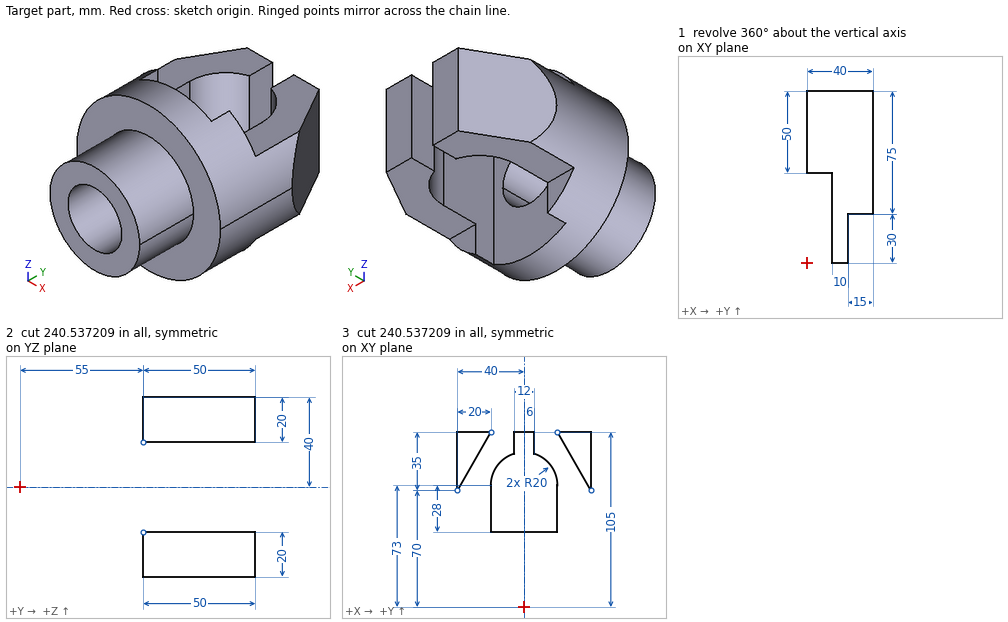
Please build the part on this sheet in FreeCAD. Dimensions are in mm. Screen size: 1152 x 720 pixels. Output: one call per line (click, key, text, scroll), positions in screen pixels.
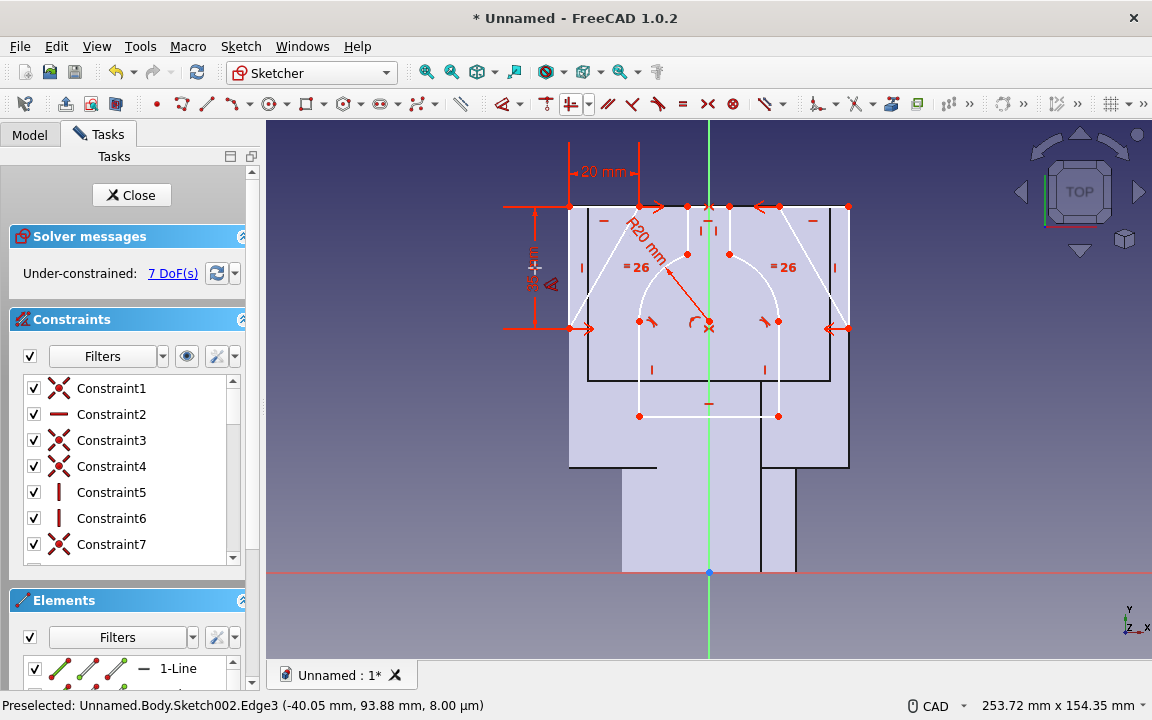
click(709, 207)
click(694, 173)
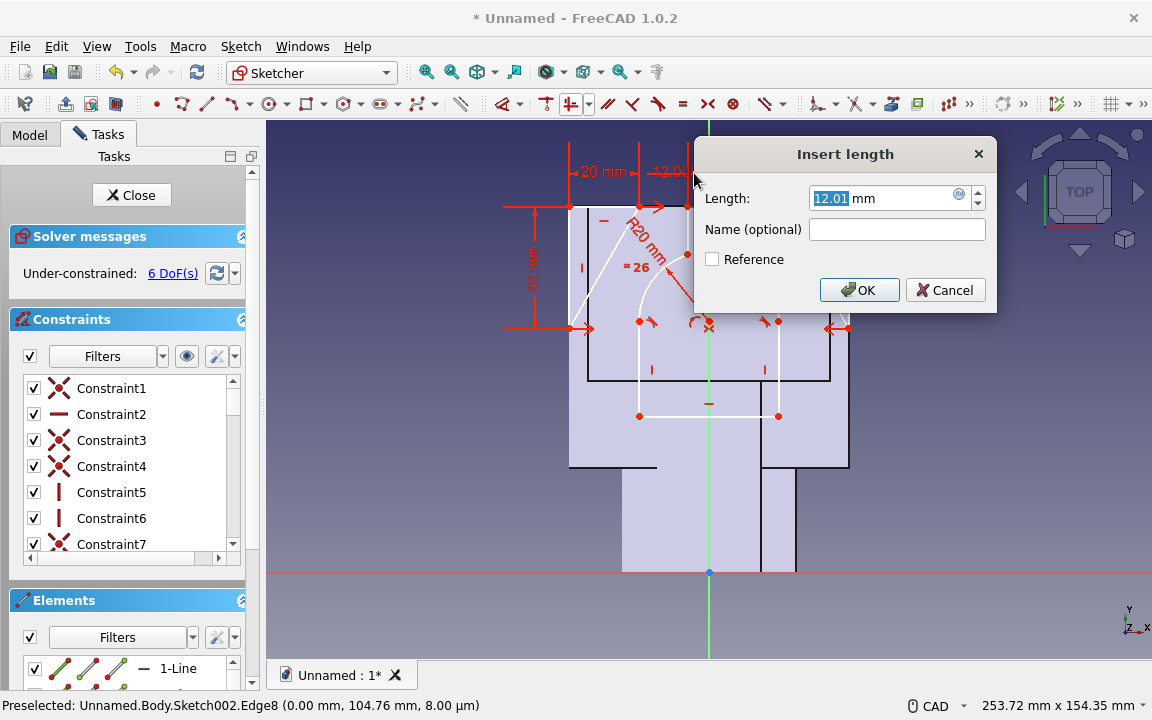
text(12)
key(Return)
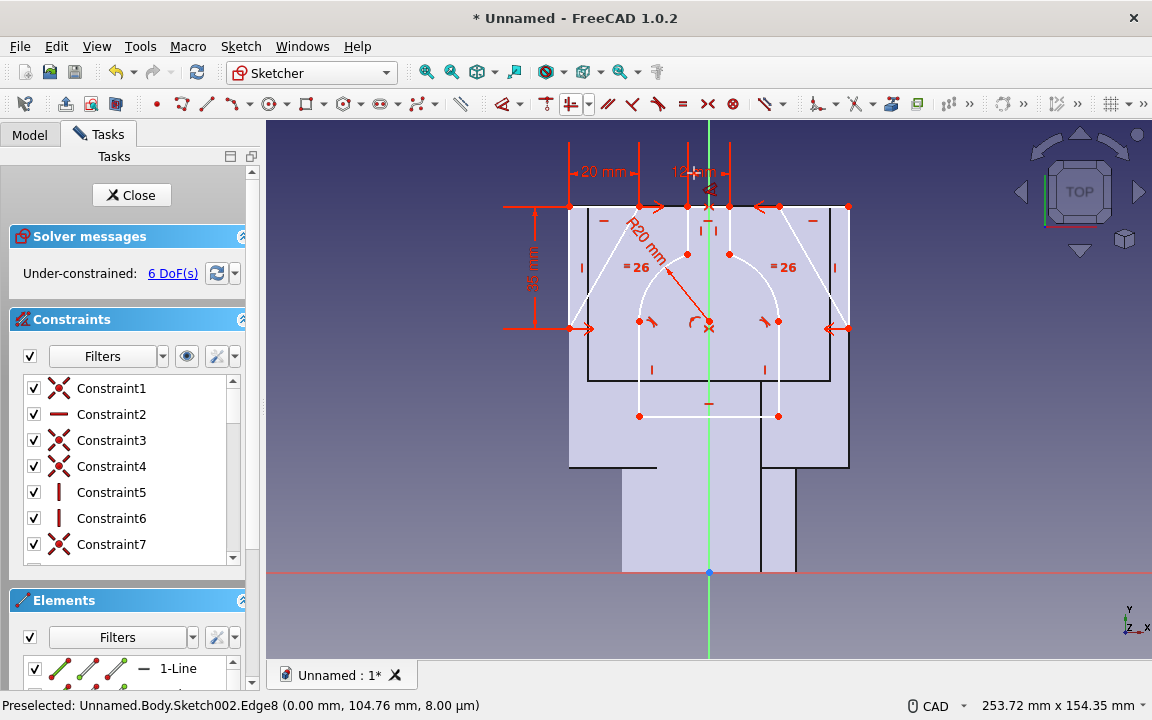
click(639, 350)
click(605, 369)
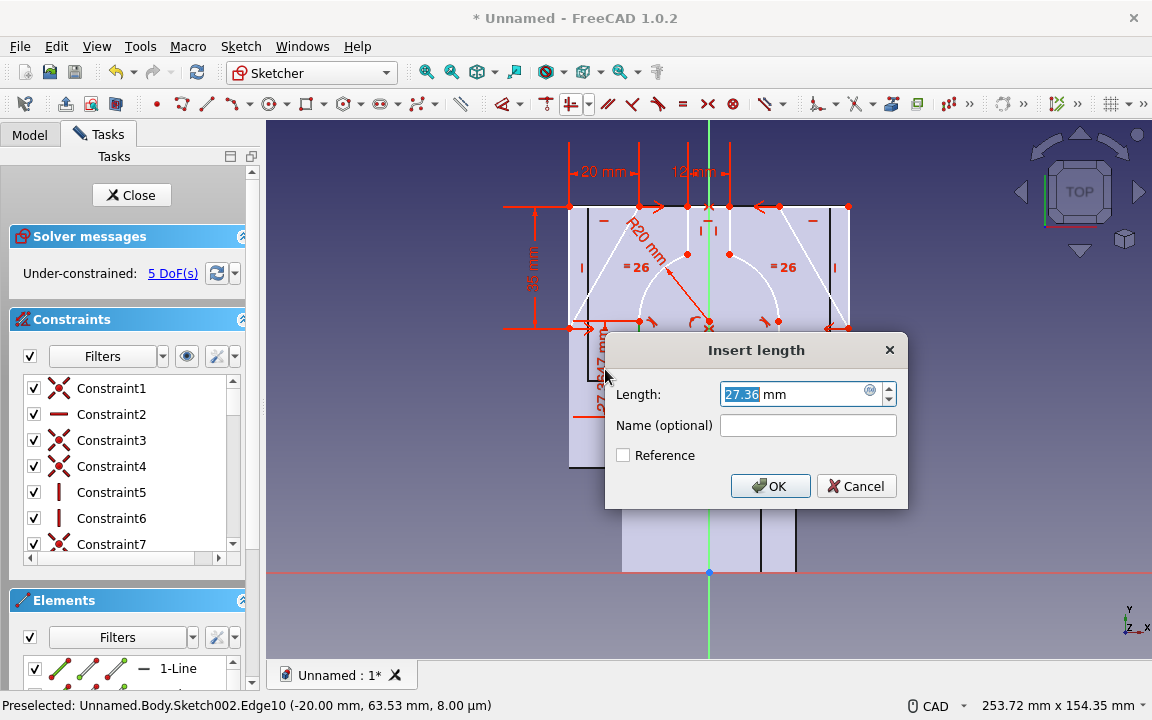
text(28)
key(Return)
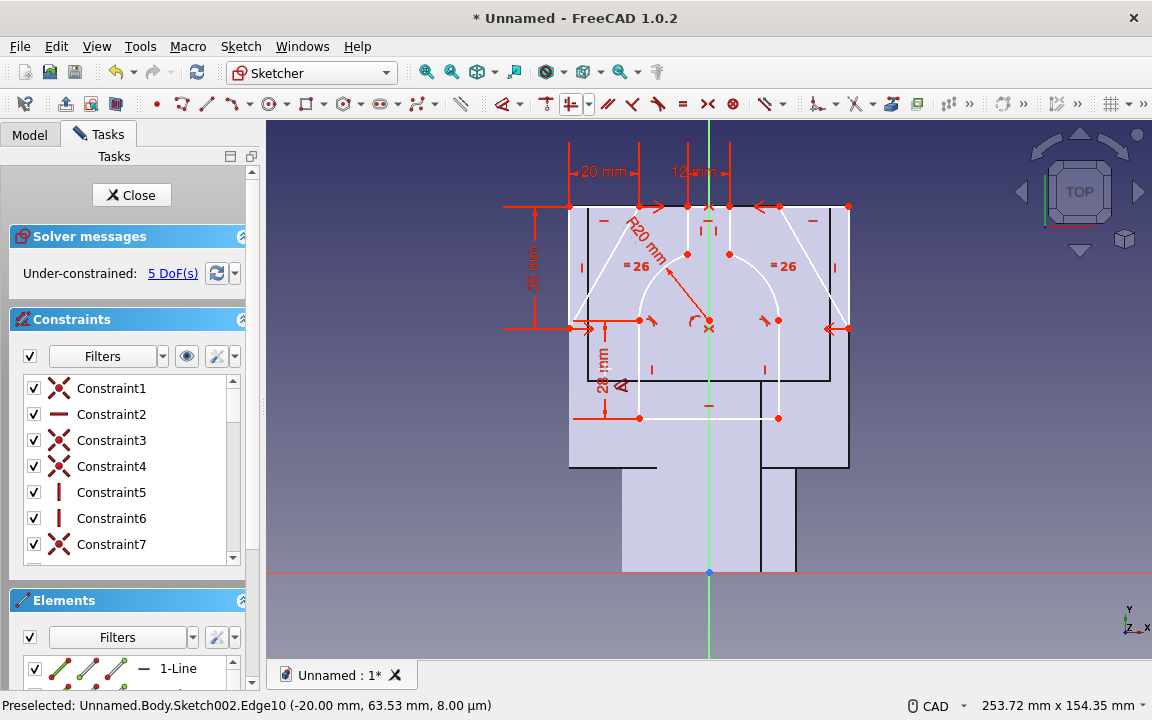
scroll(730, 254, up, 4)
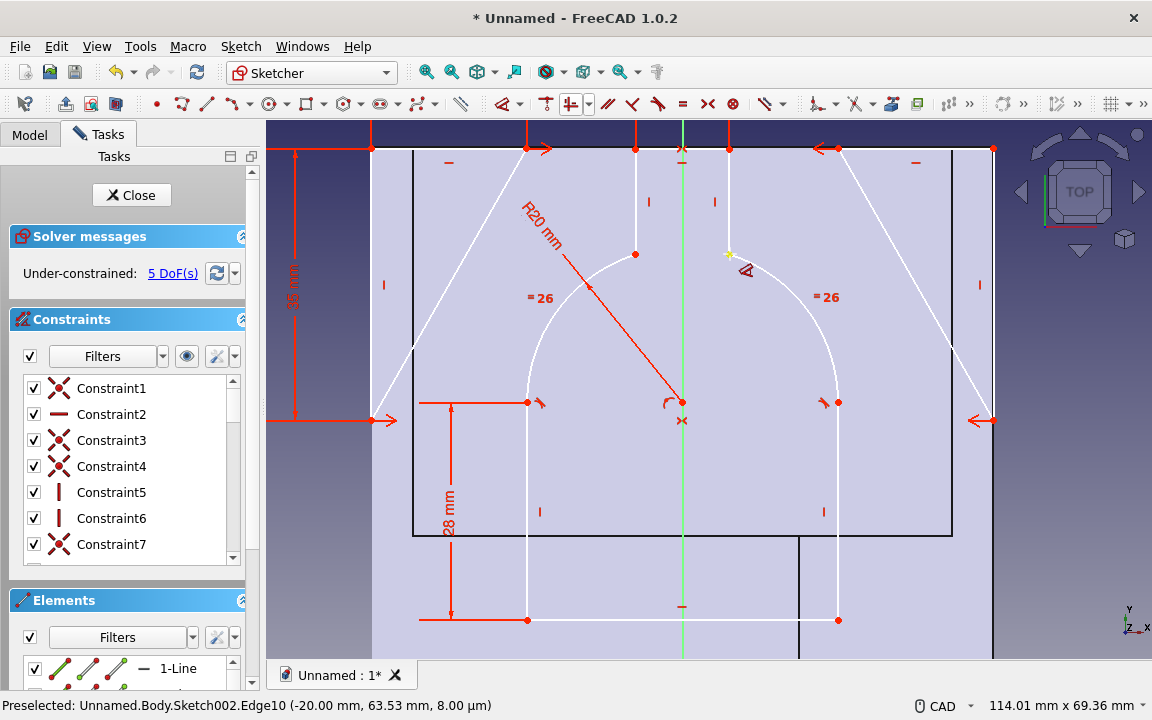
click(729, 254)
click(706, 220)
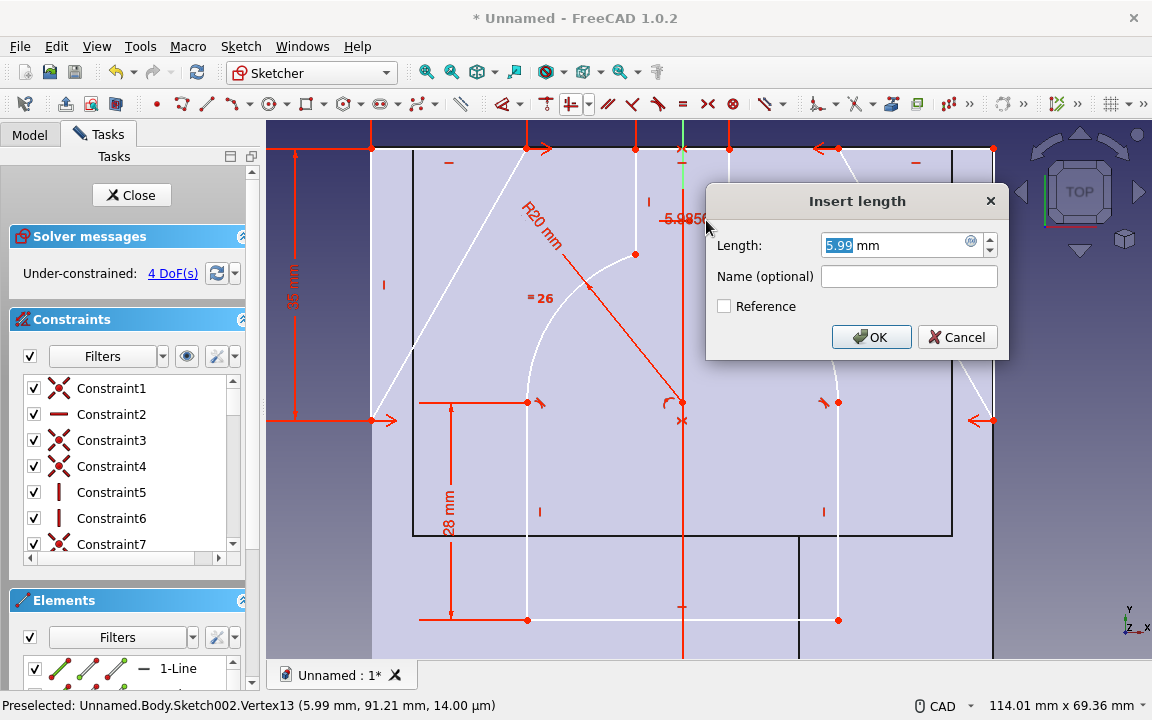
text(6)
key(Return)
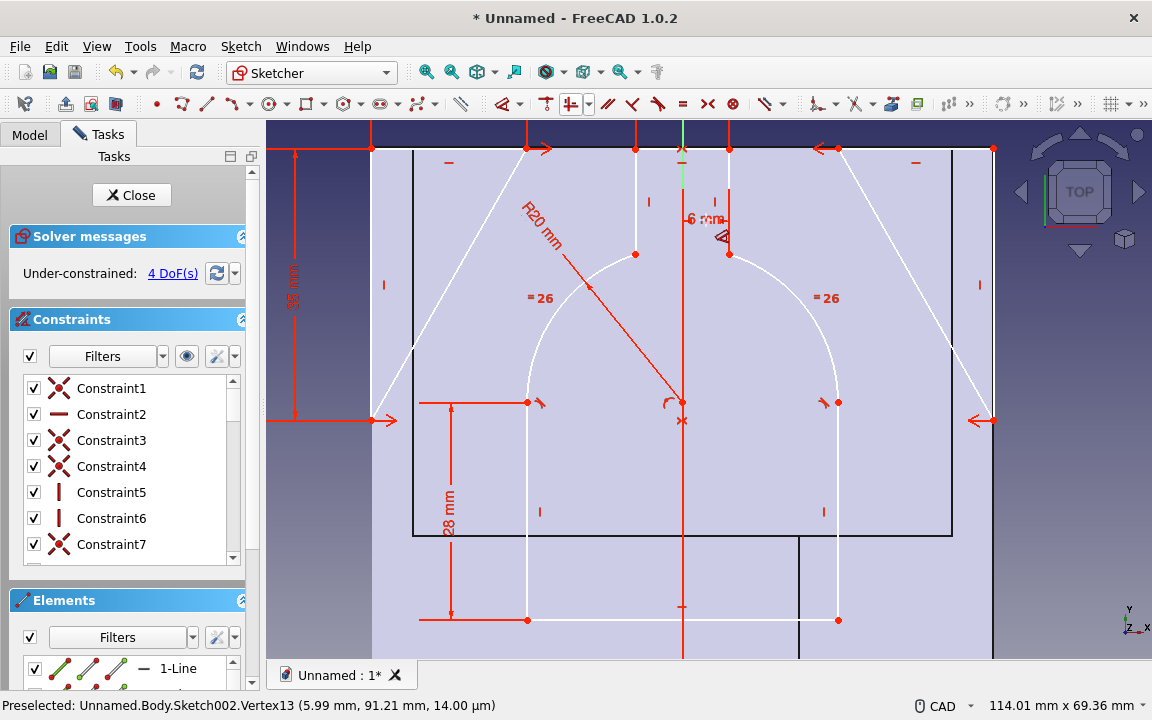
click(371, 421)
click(455, 387)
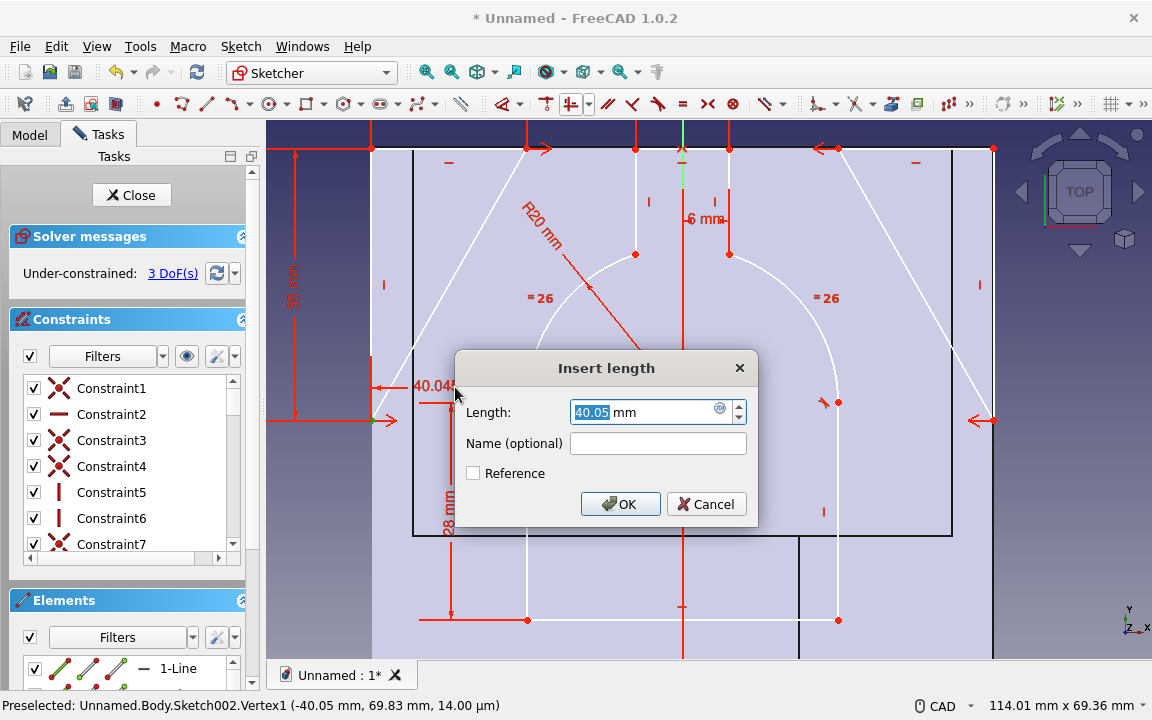
text(40)
key(Return)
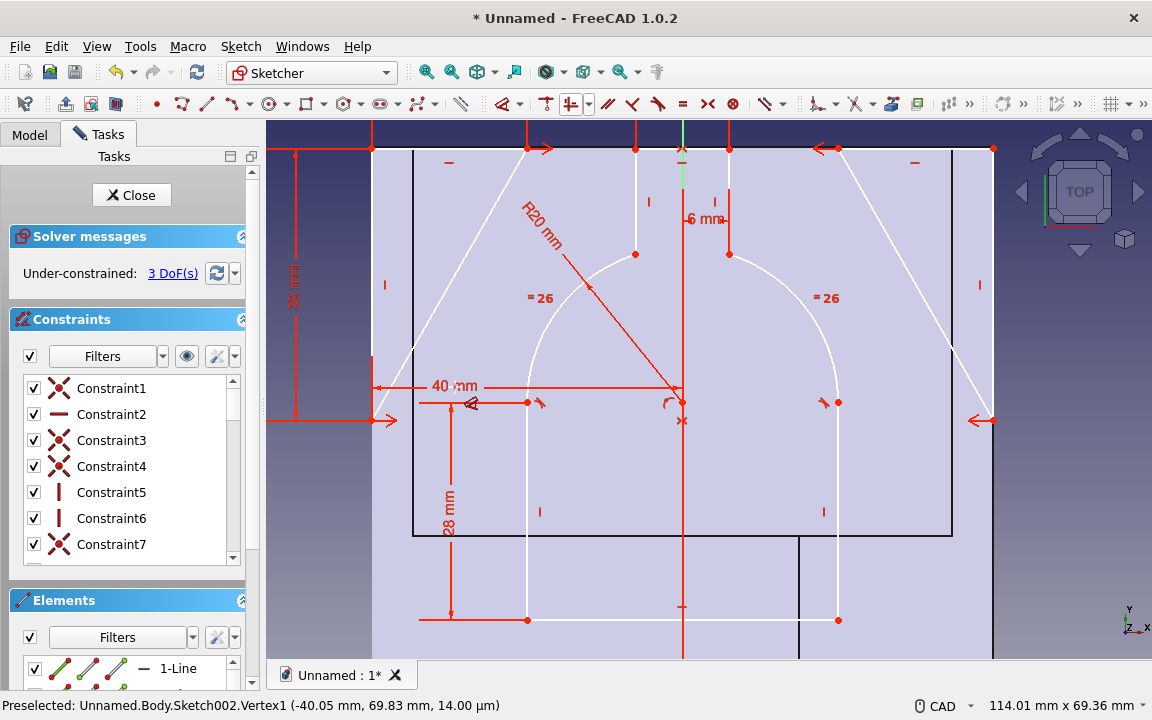
click(372, 421)
click(338, 526)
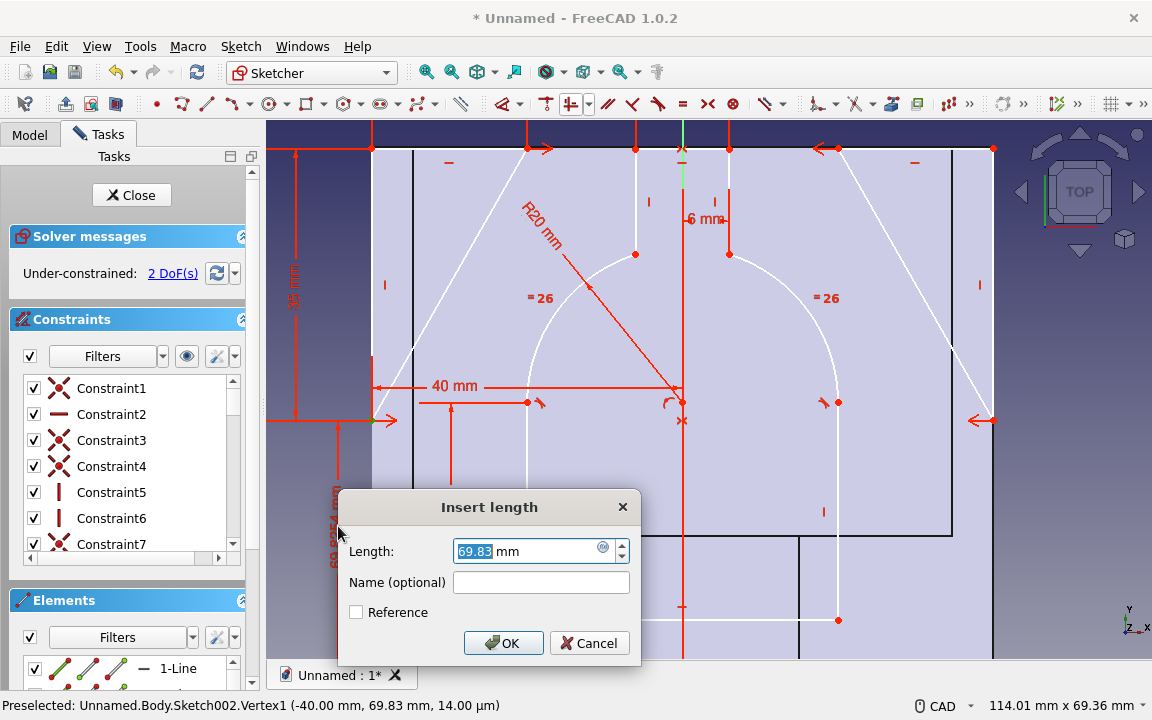
text(70)
key(Return)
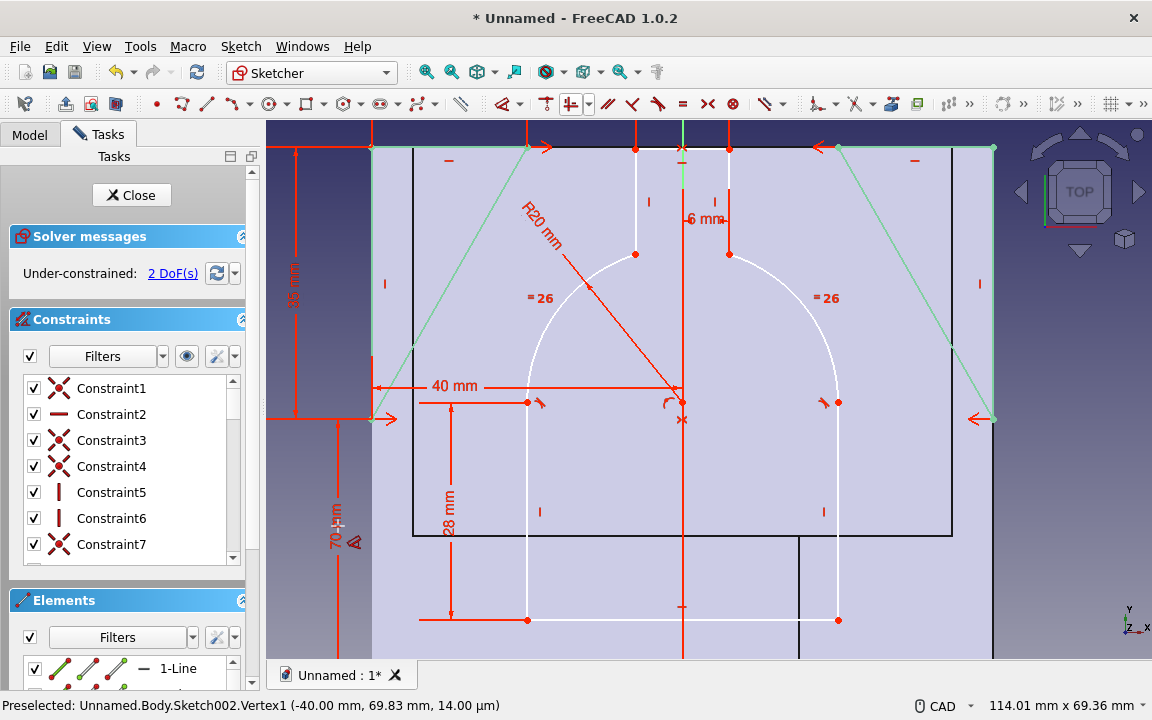
click(527, 403)
click(493, 464)